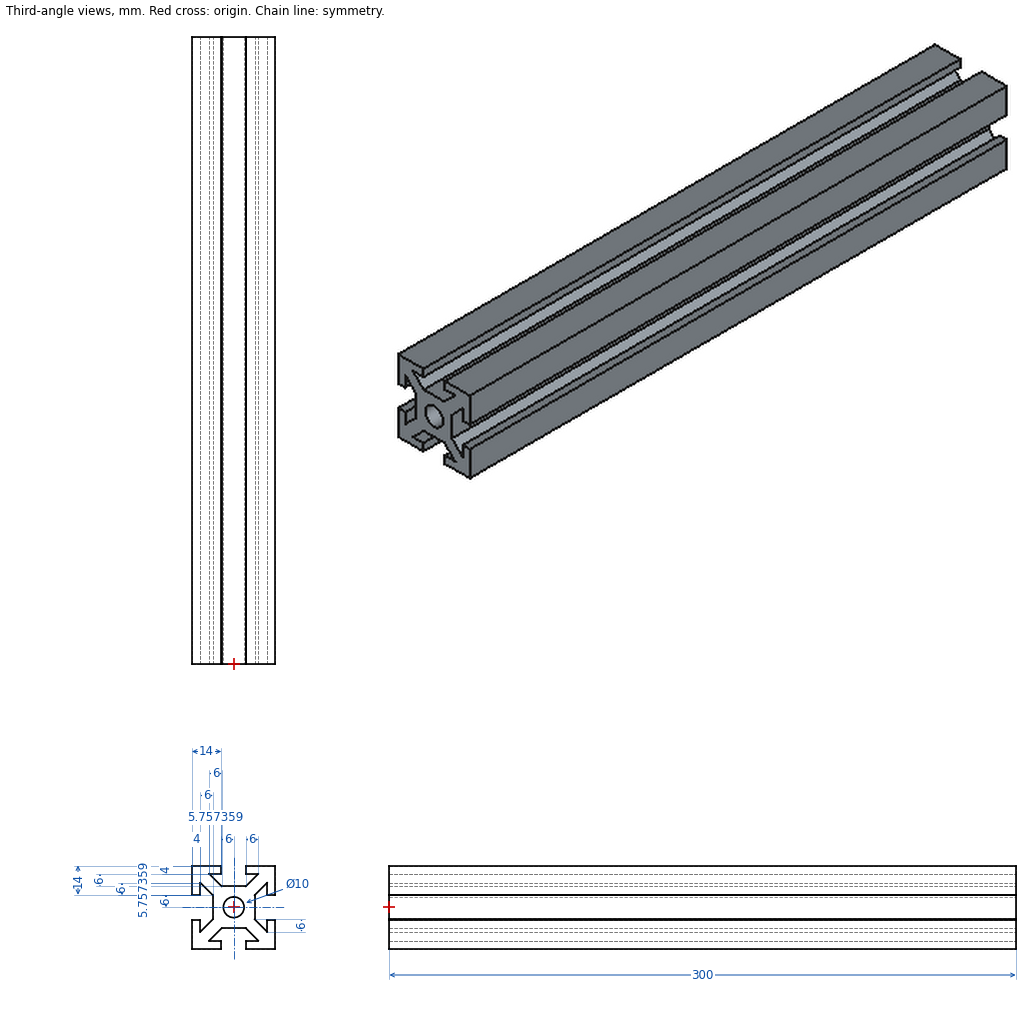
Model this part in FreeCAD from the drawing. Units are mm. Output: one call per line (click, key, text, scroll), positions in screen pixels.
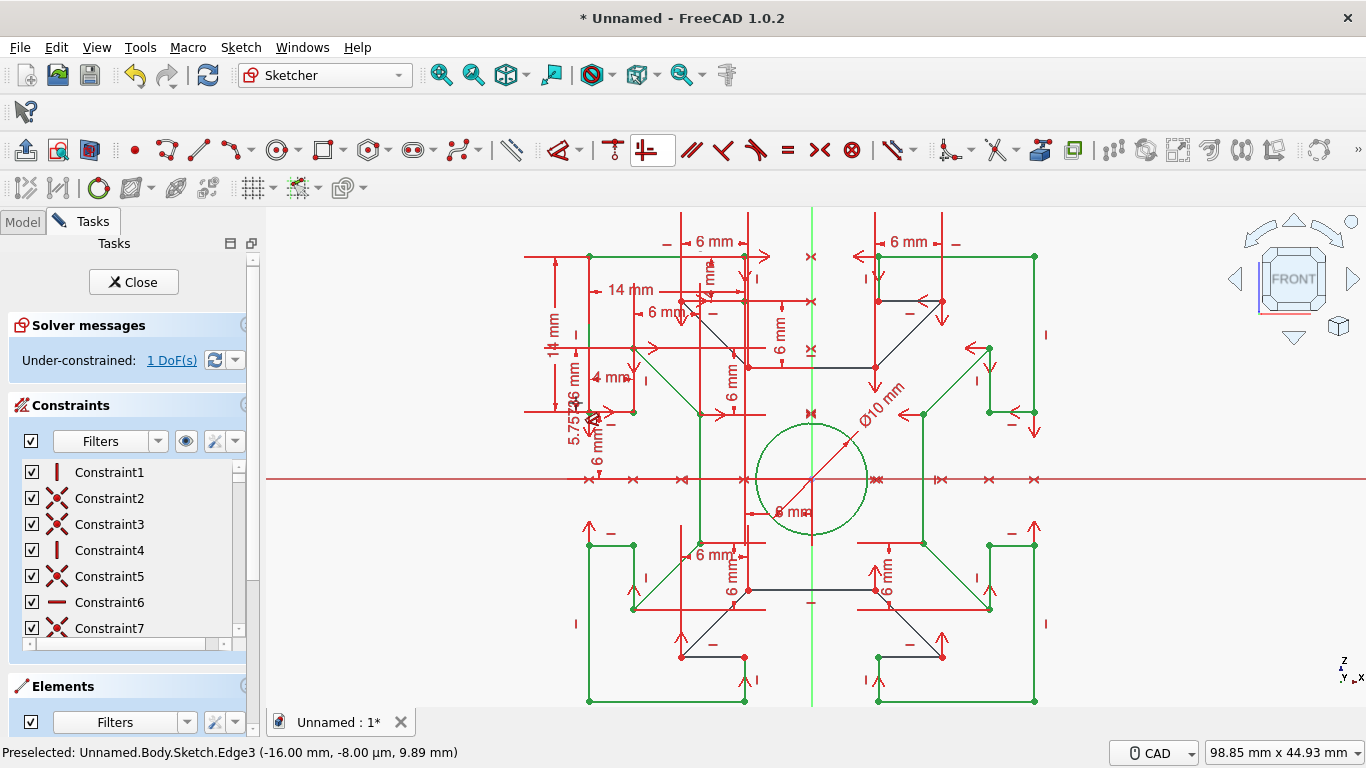
click(726, 301)
click(691, 335)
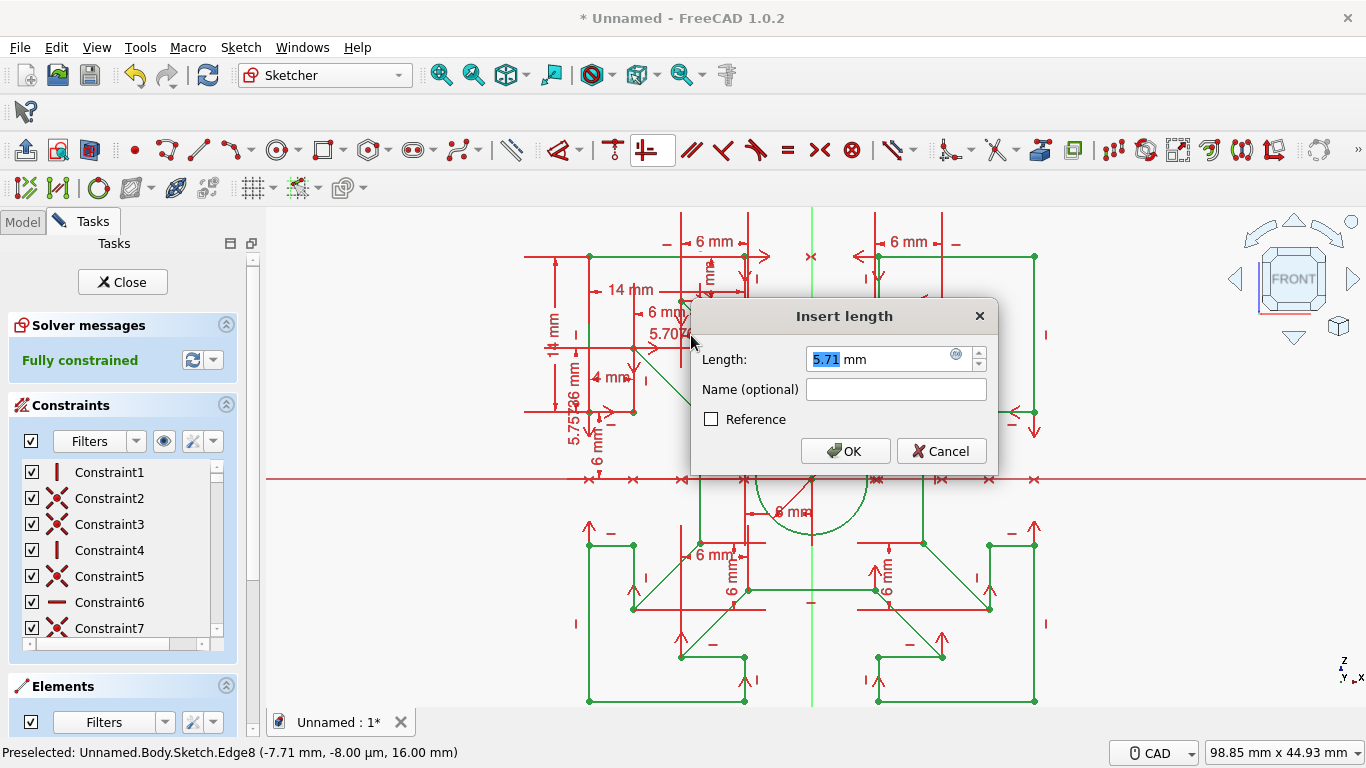
text(5.757359)
key(Return)
key(Escape)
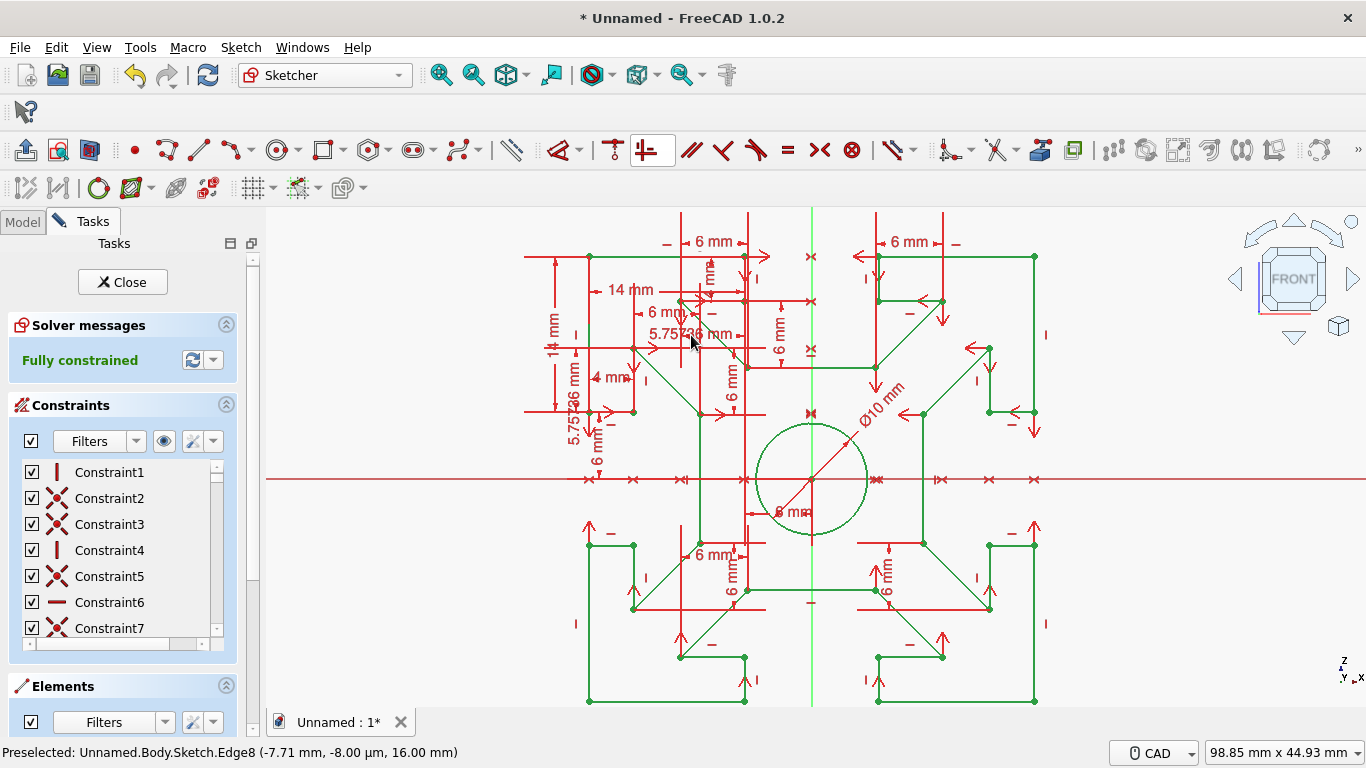
click(123, 282)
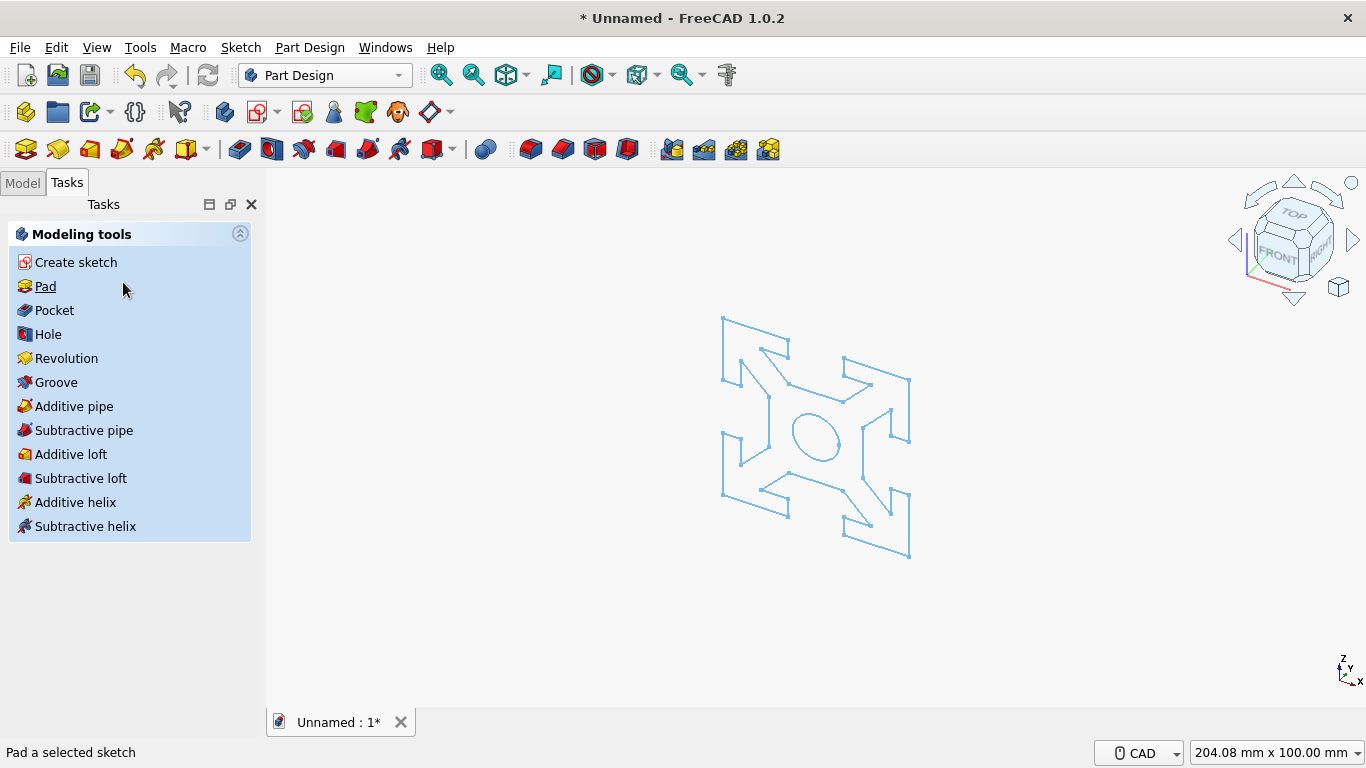
click(26, 150)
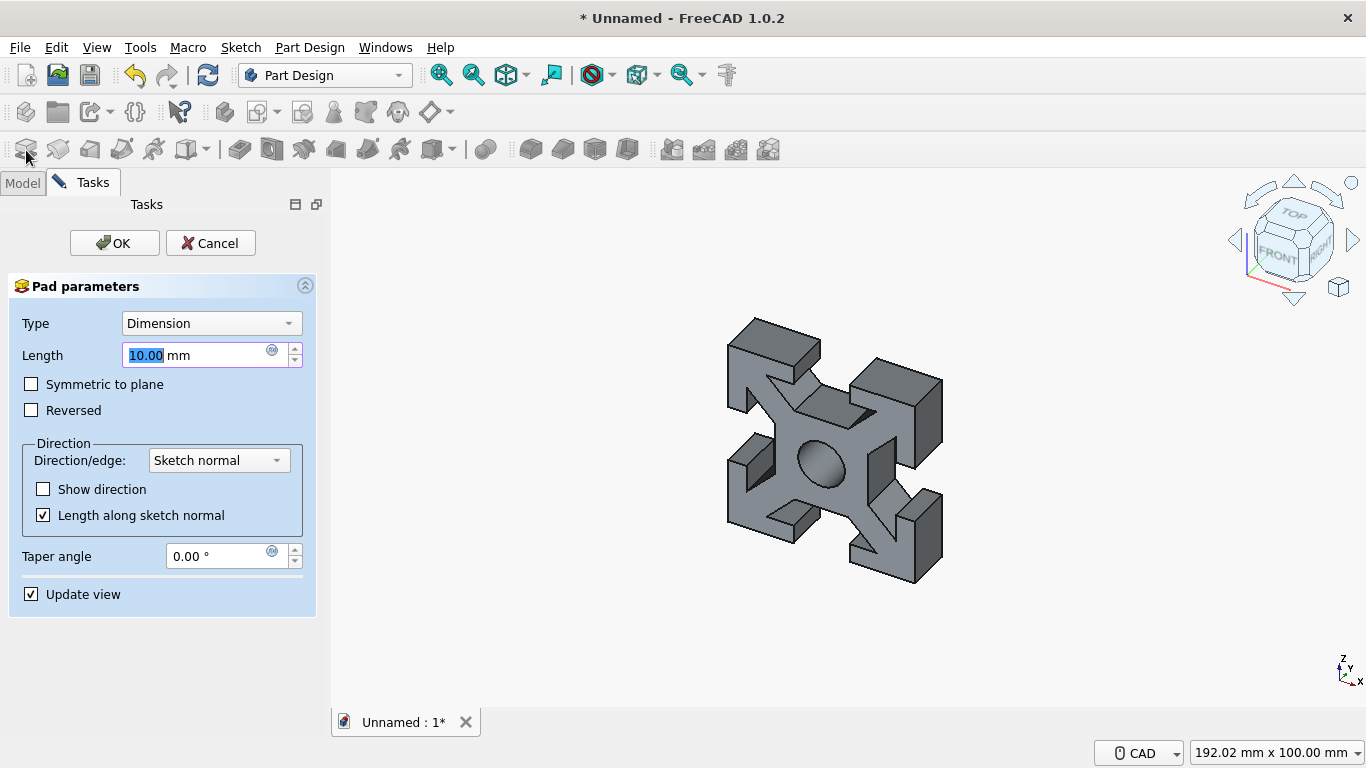
text(300)
key(Tab)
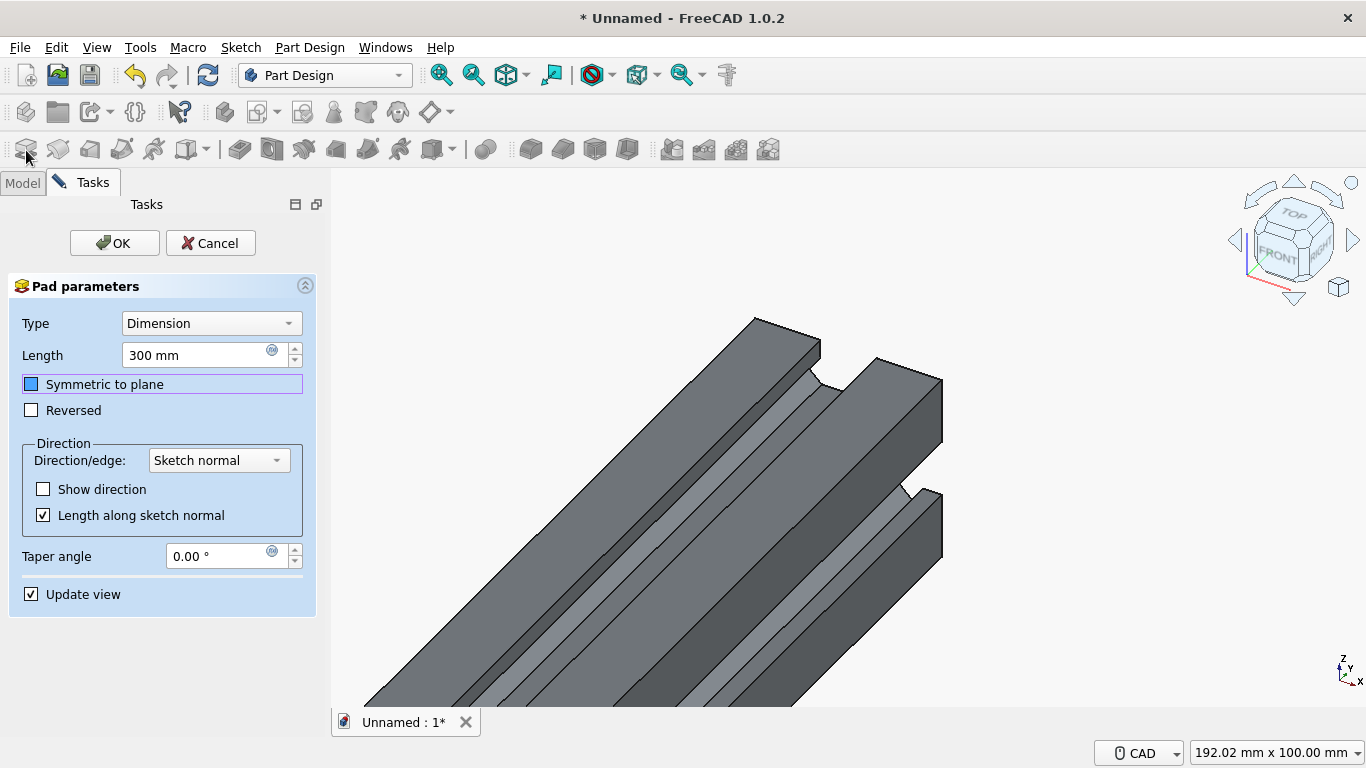
click(30, 410)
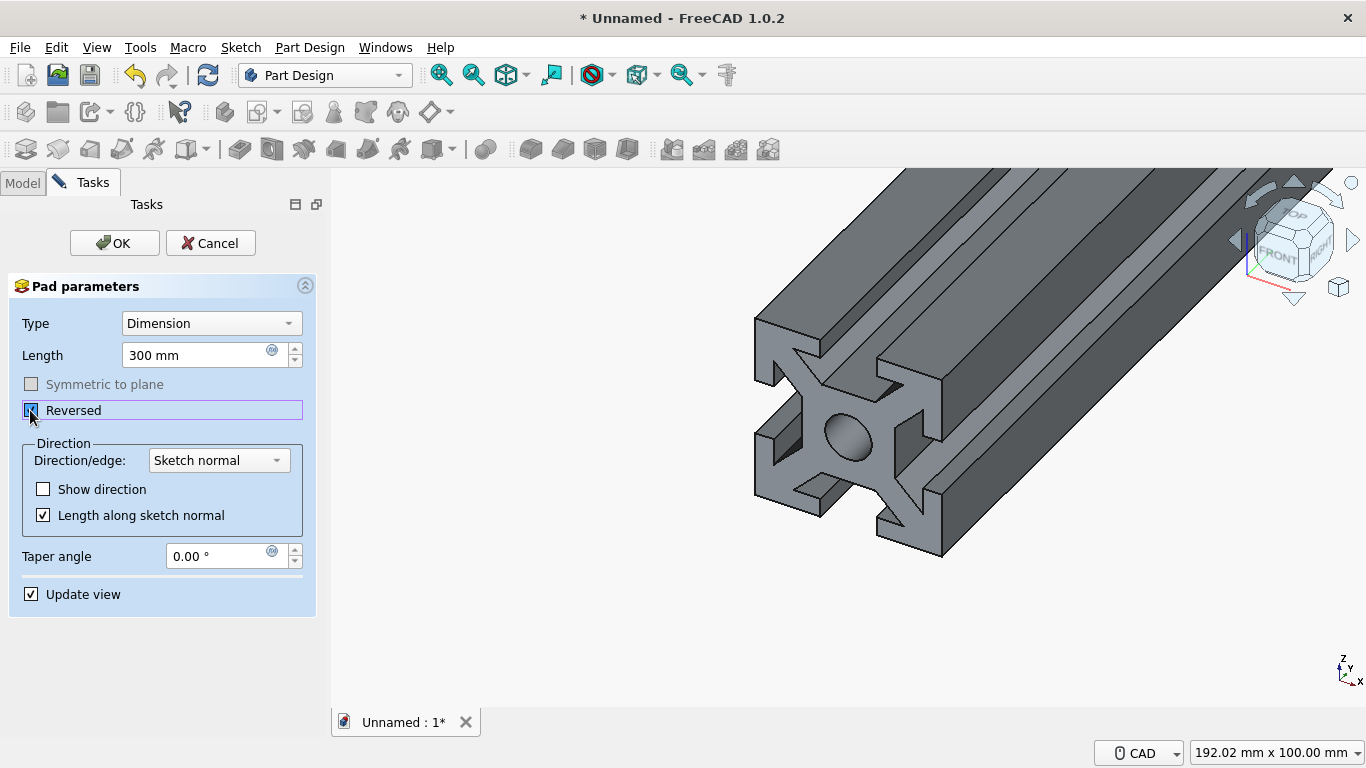
click(115, 243)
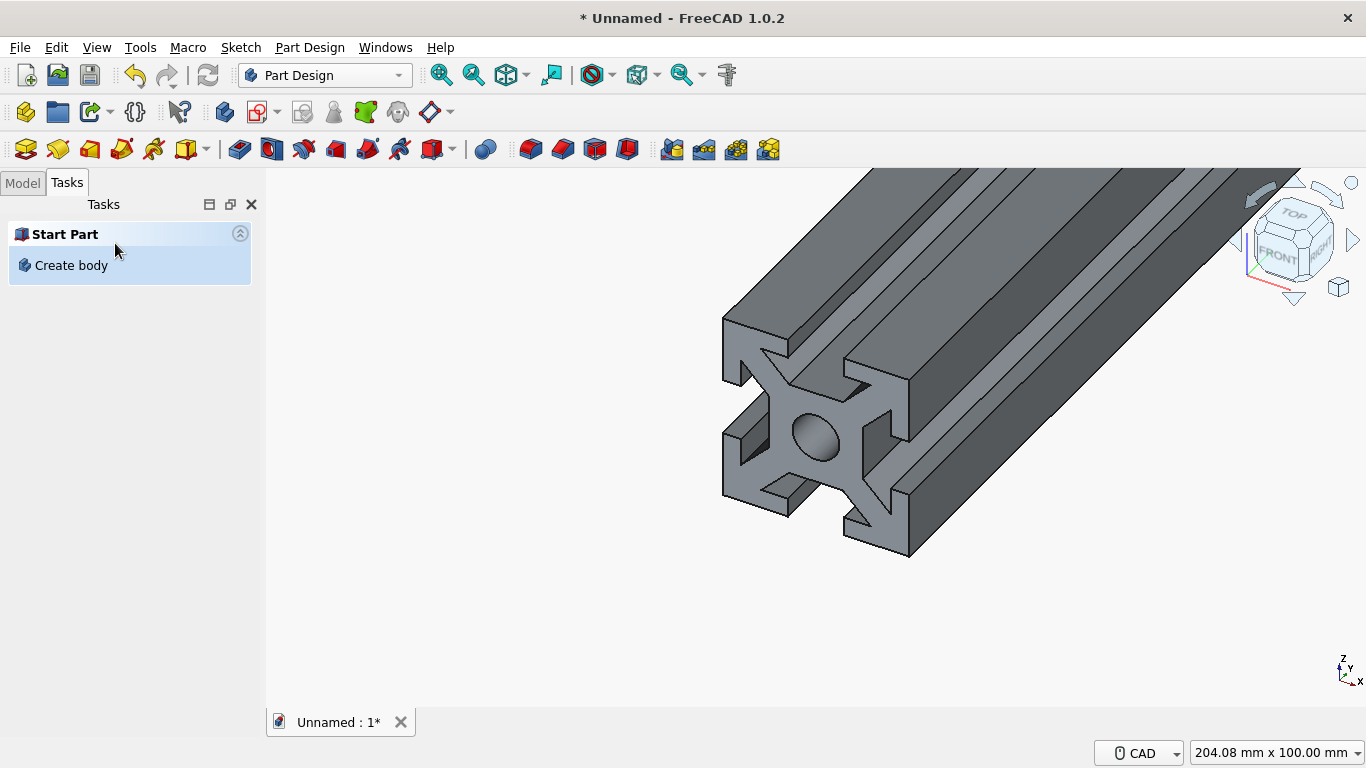
key(0)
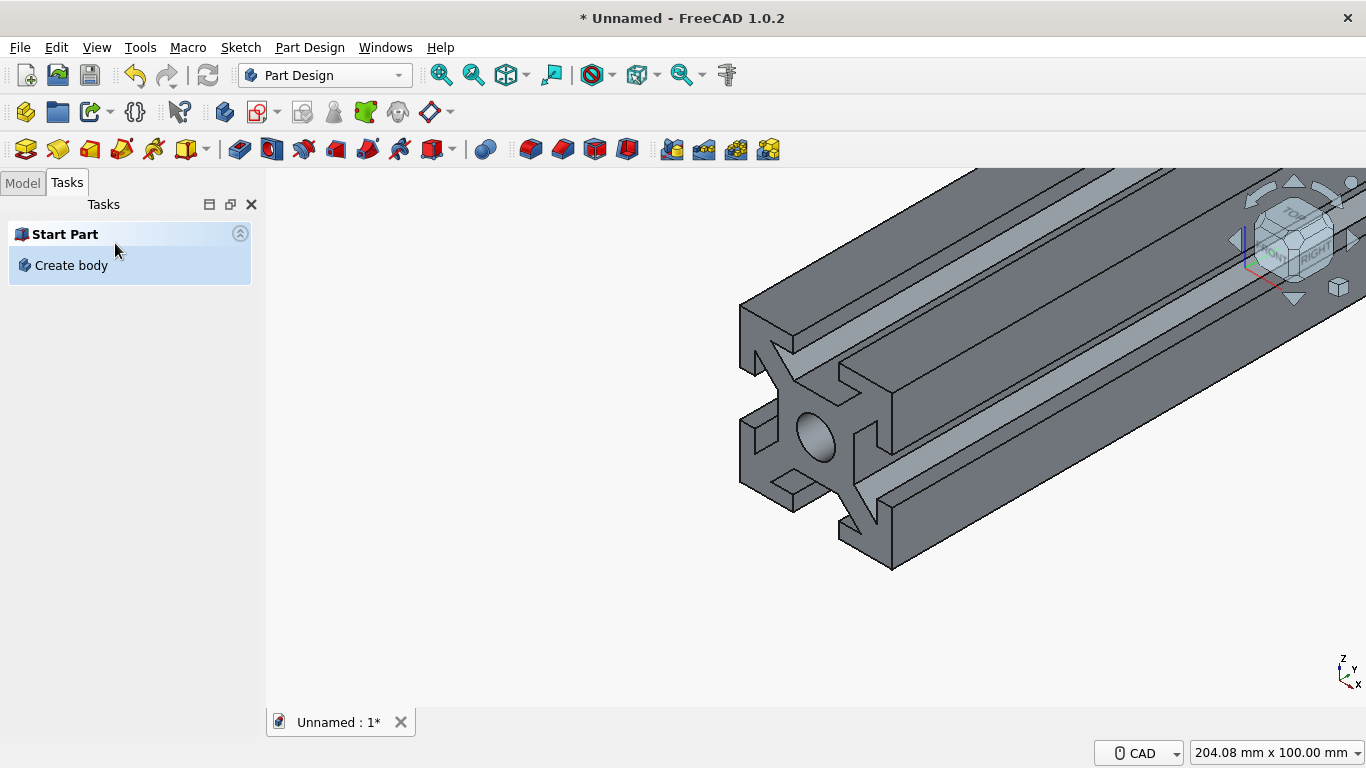
click(442, 76)